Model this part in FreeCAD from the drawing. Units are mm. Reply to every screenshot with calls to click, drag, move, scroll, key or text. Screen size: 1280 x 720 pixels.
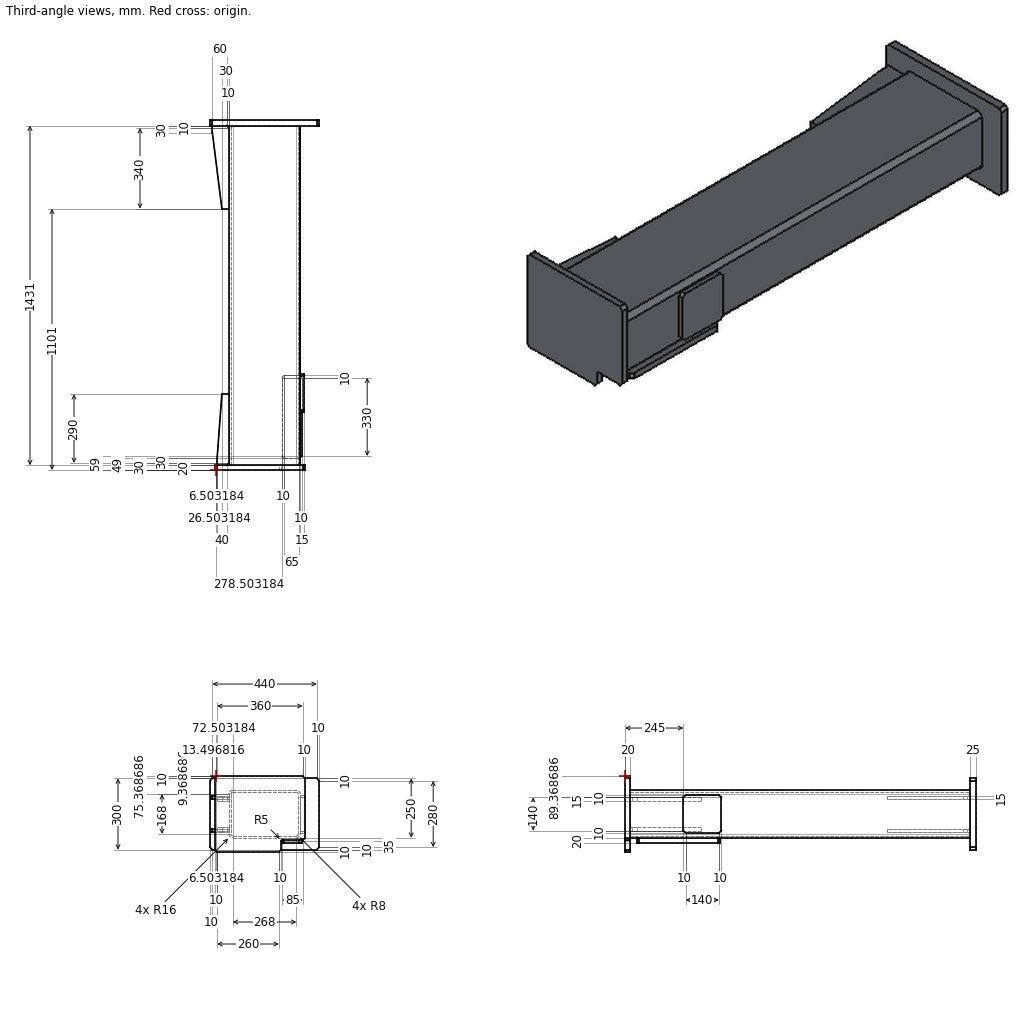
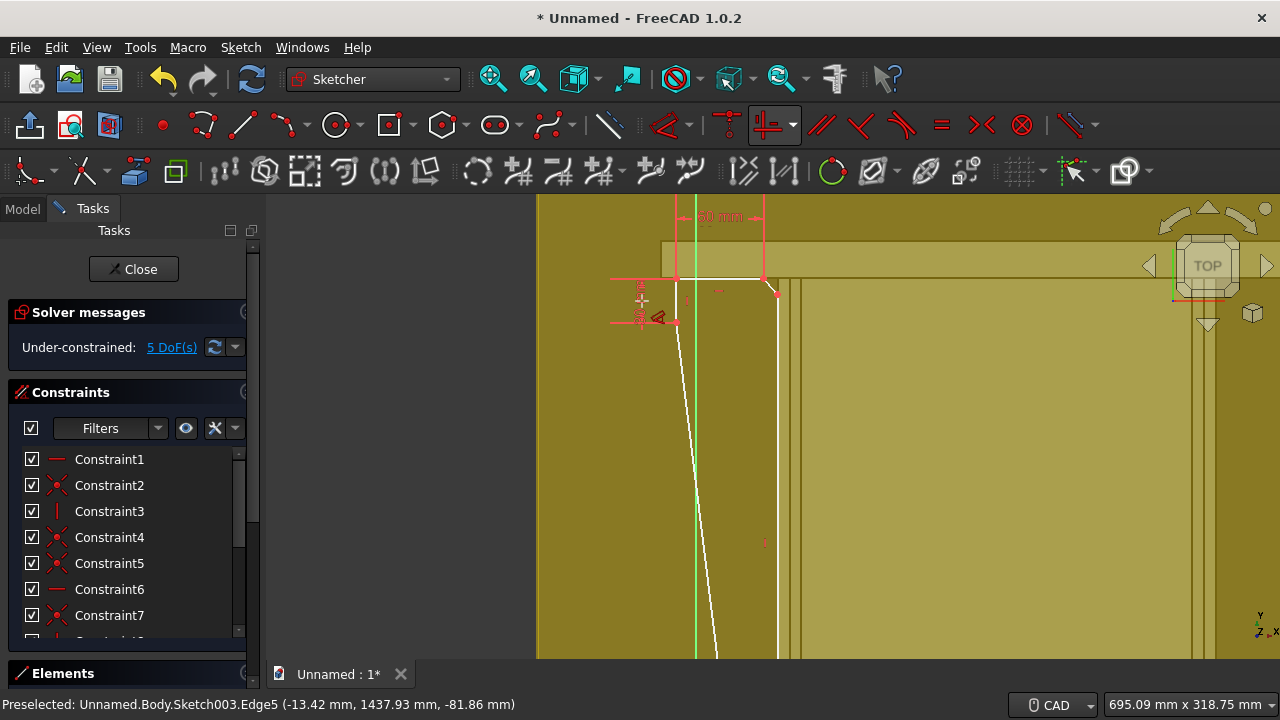
click(778, 444)
click(812, 463)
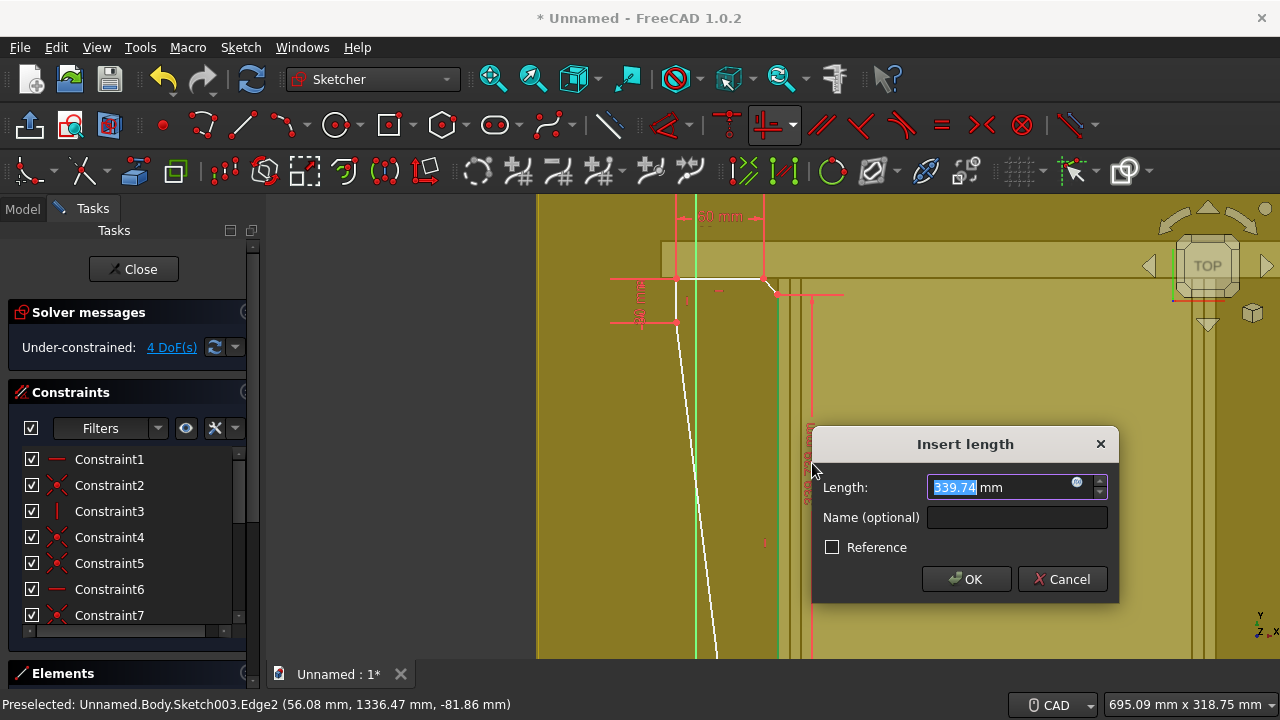
text(340)
key(Return)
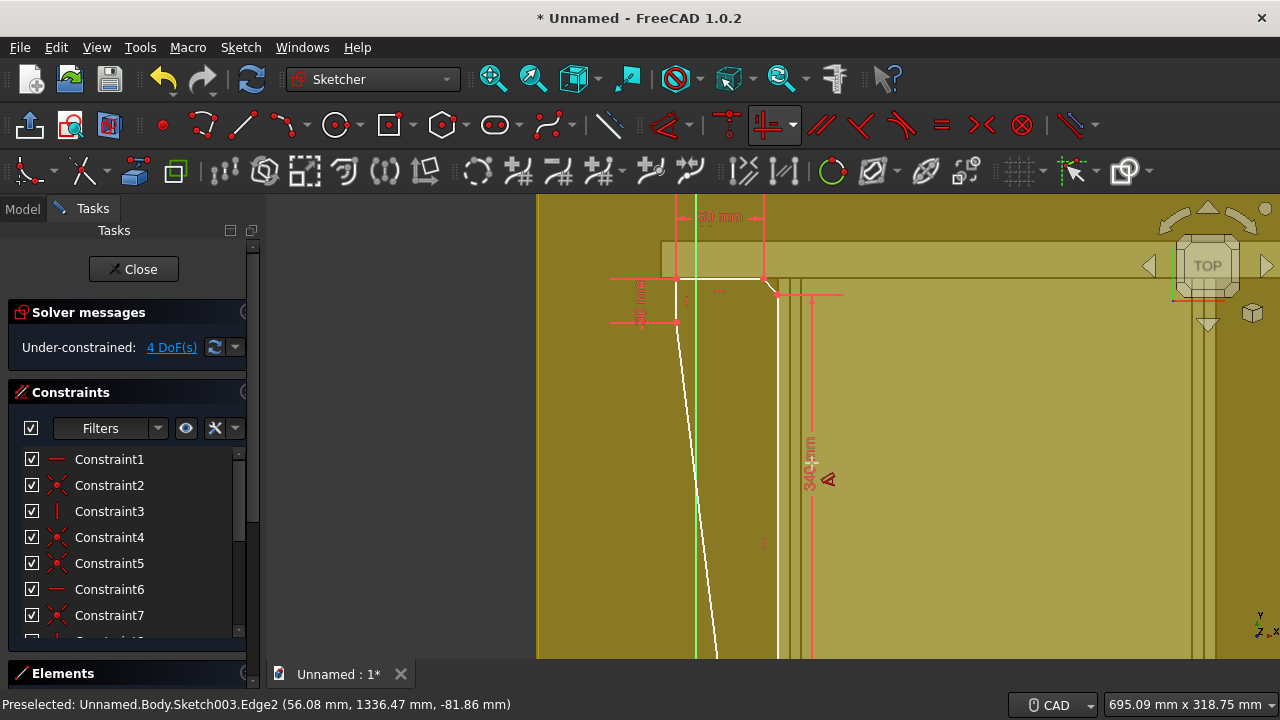
scroll(771, 287, up, 6)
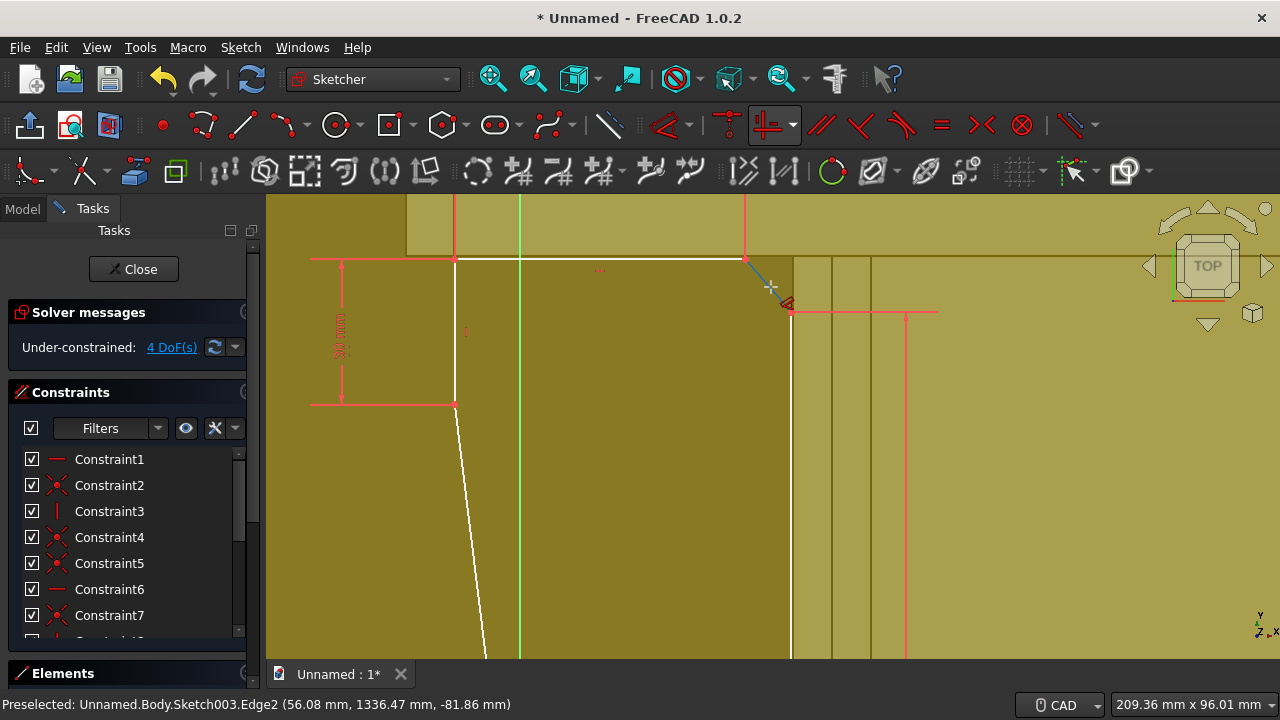
click(768, 286)
click(768, 225)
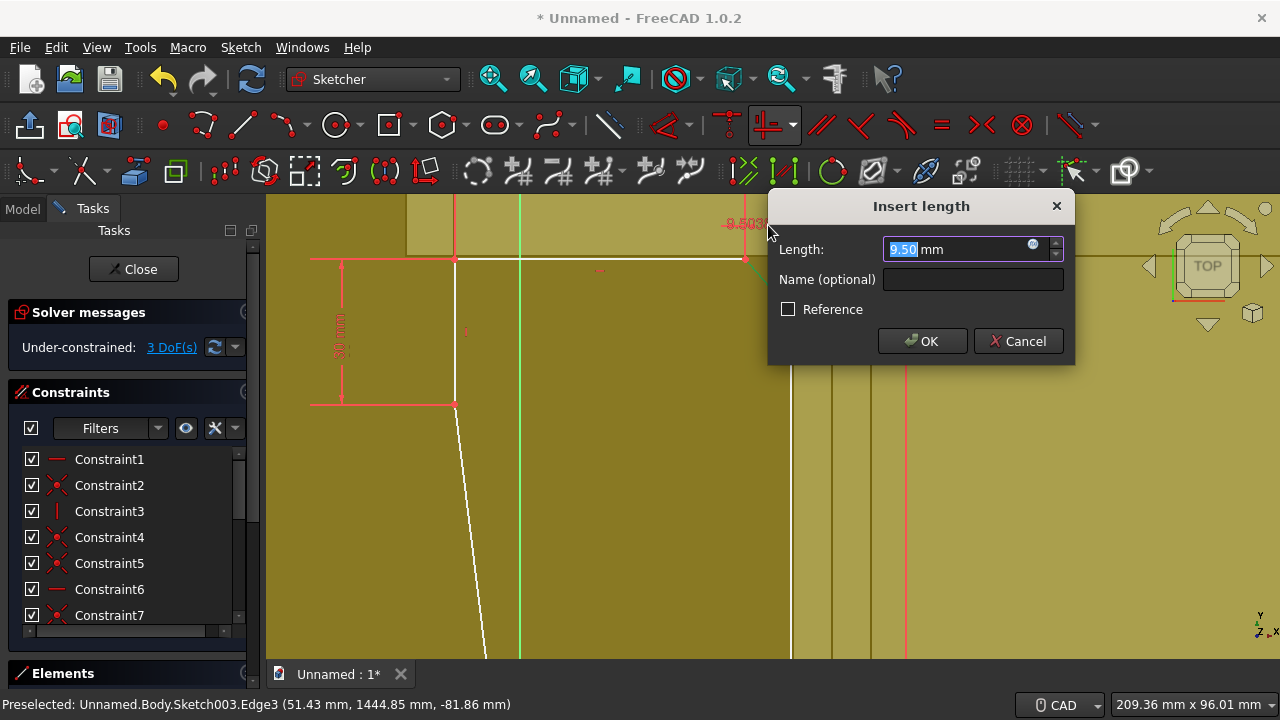
text(10)
key(Return)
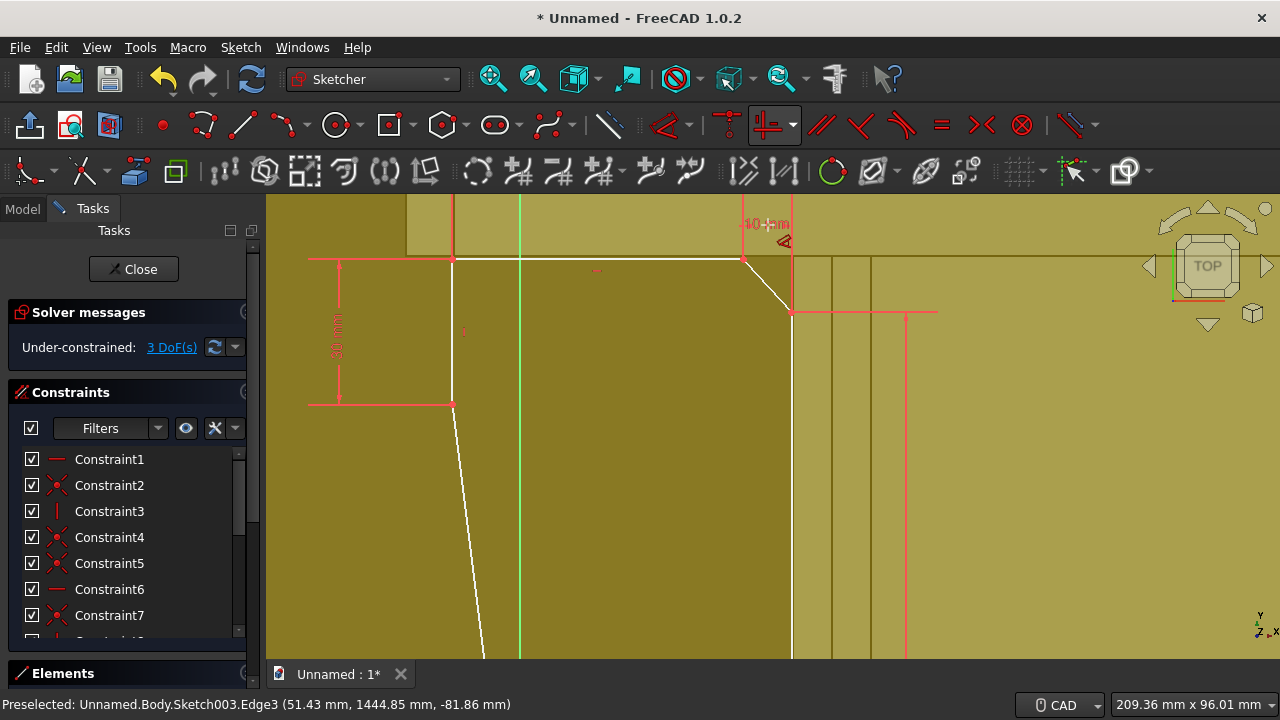
click(777, 296)
click(826, 286)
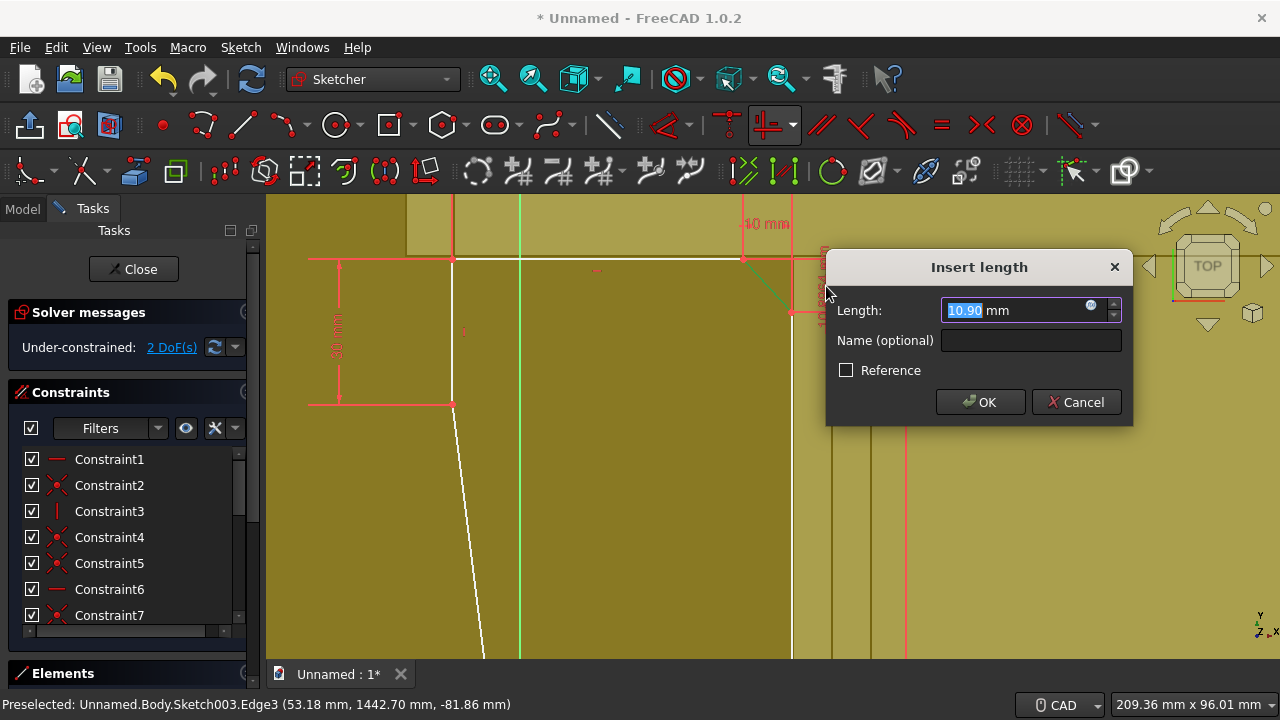
text(10)
key(Return)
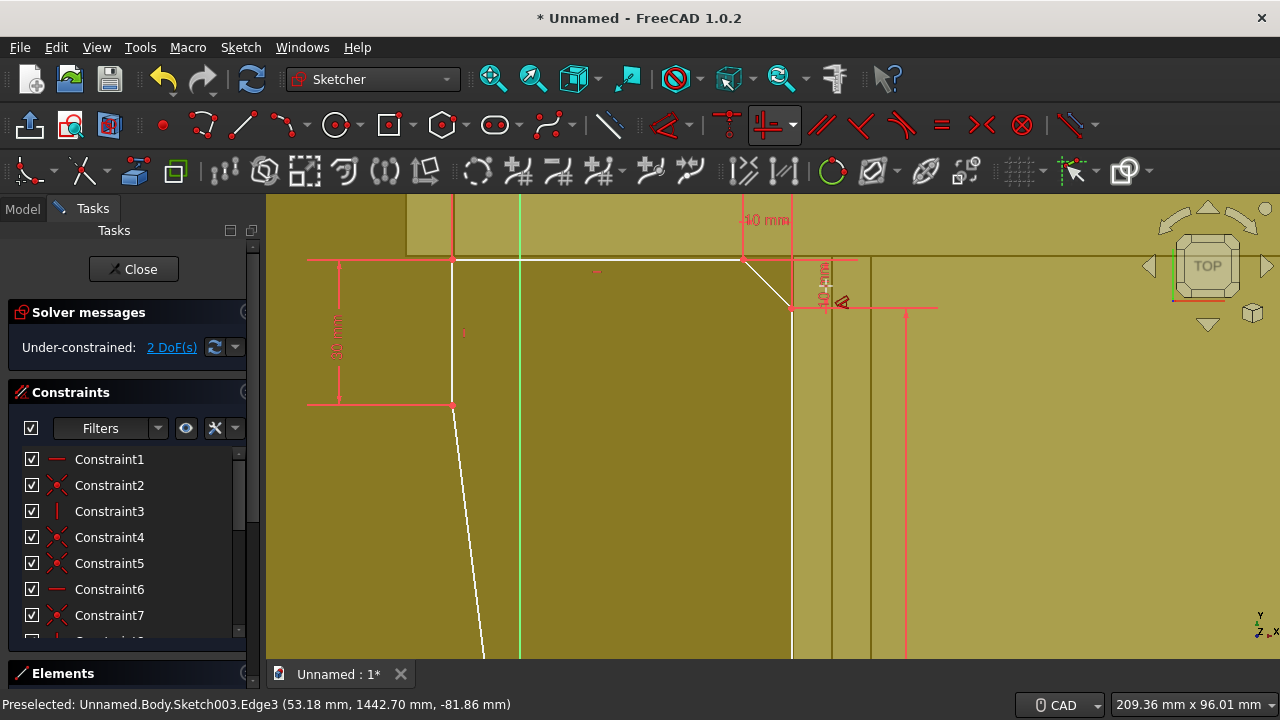
scroll(720, 292, down, 9)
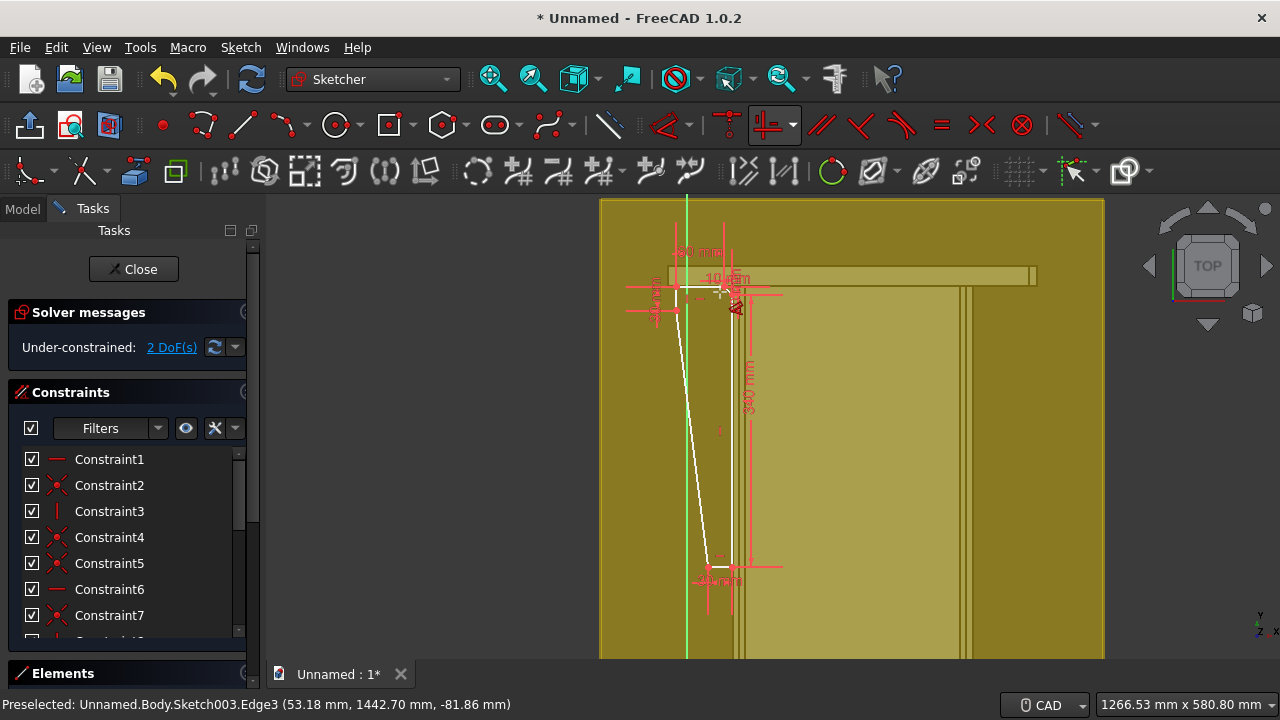
click(708, 567)
click(653, 614)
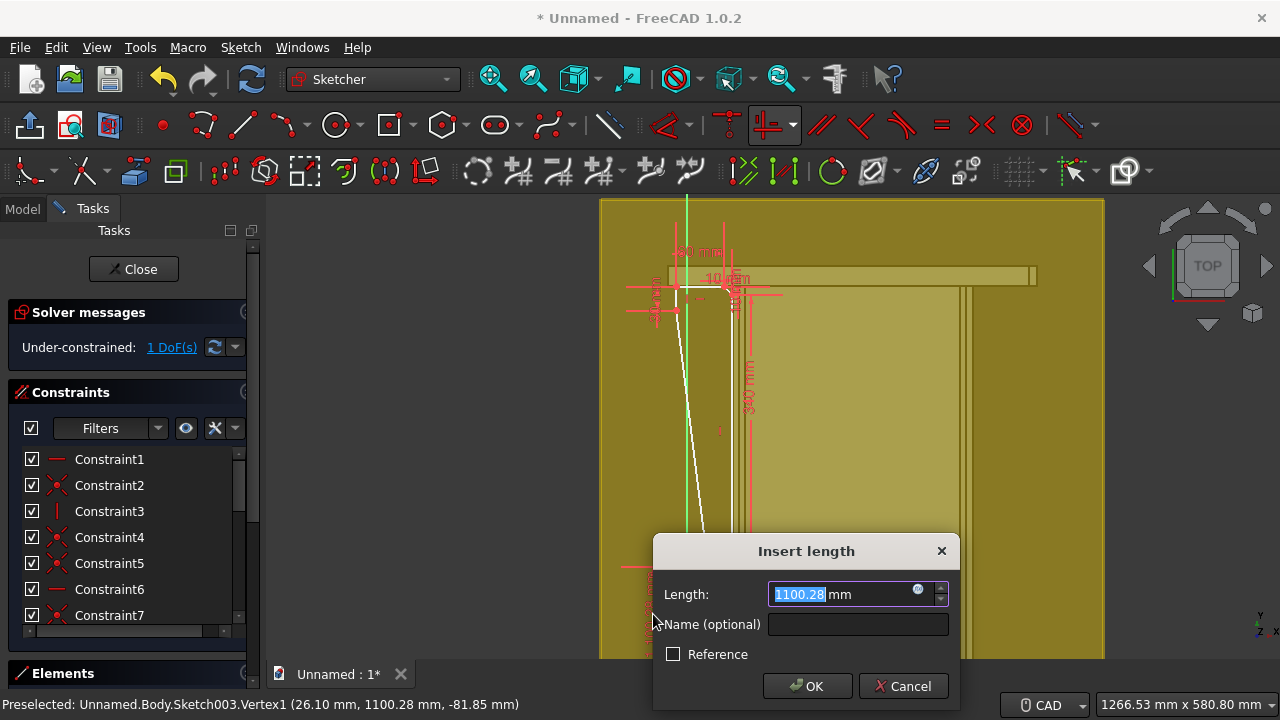
text(1101)
key(Return)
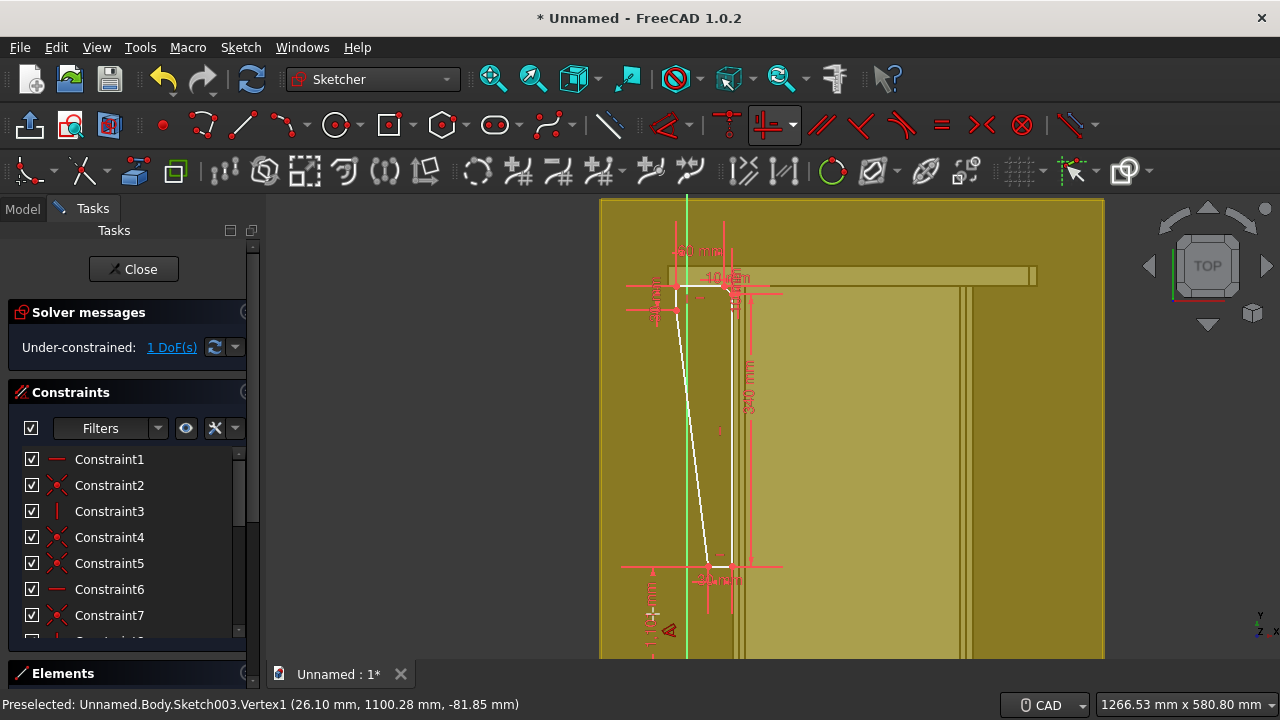
scroll(708, 567, up, 4)